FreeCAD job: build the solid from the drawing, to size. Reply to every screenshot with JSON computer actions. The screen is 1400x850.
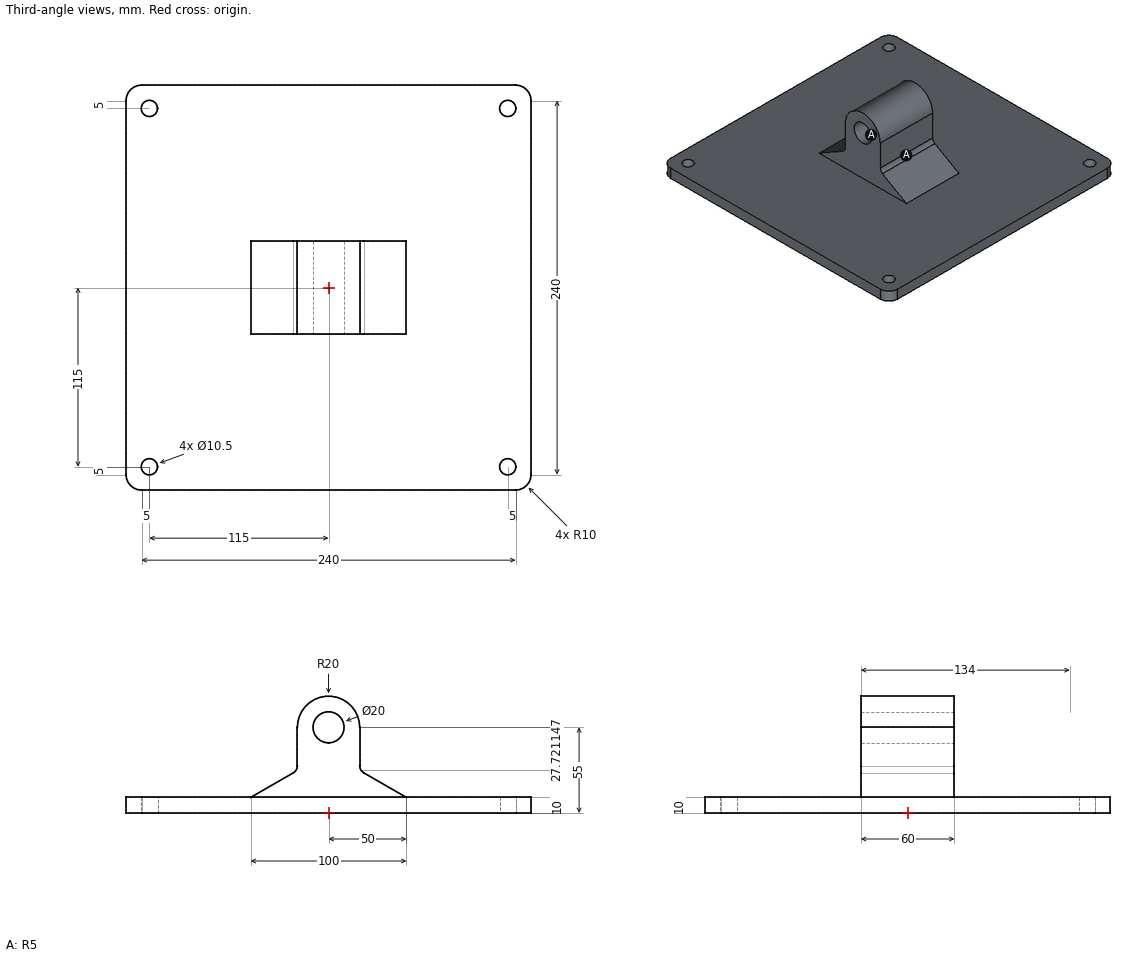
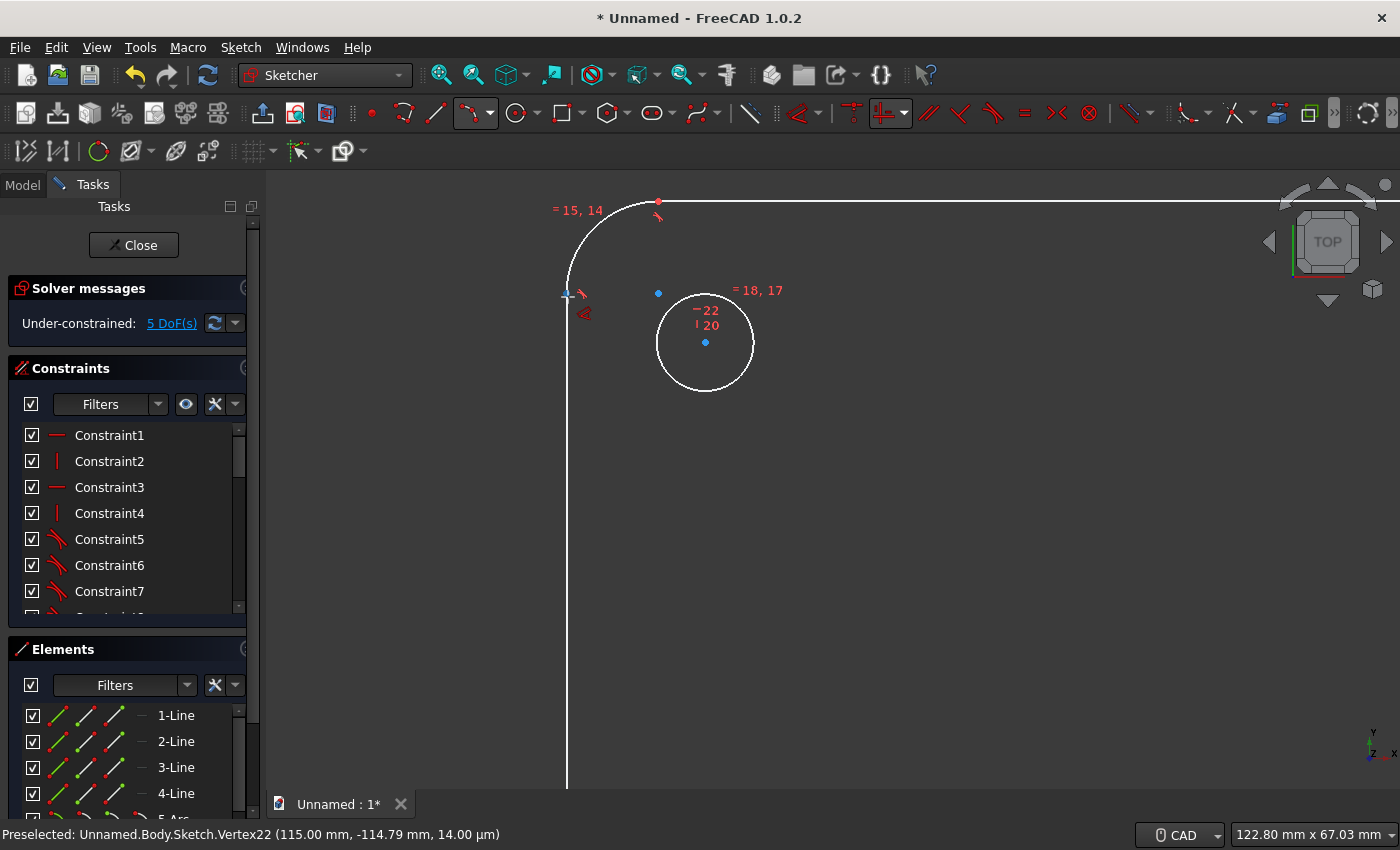
{"action": "left_click", "coordinate": [567, 294]}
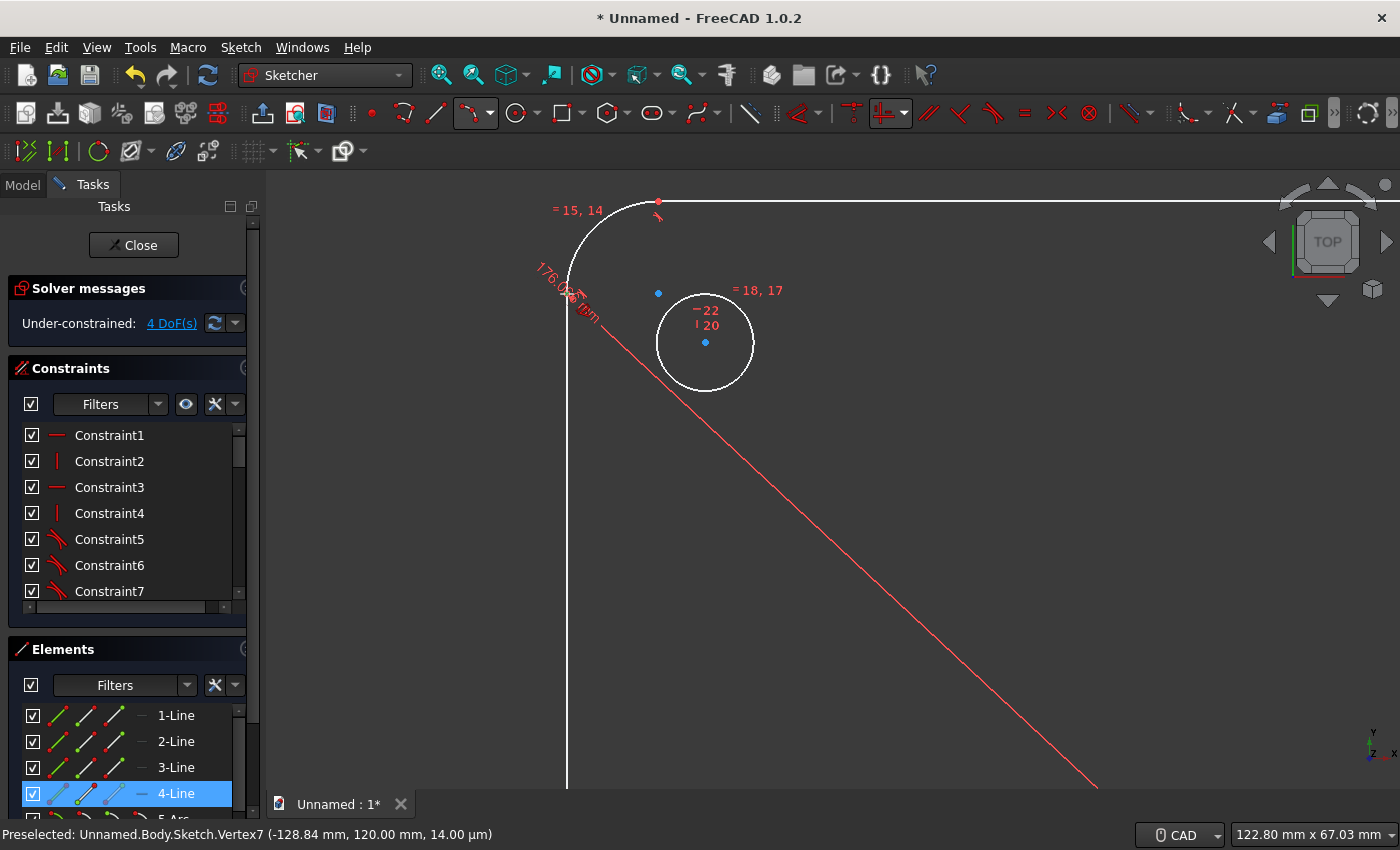
{"action": "left_click", "coordinate": [705, 343]}
{"action": "left_click", "coordinate": [533, 318]}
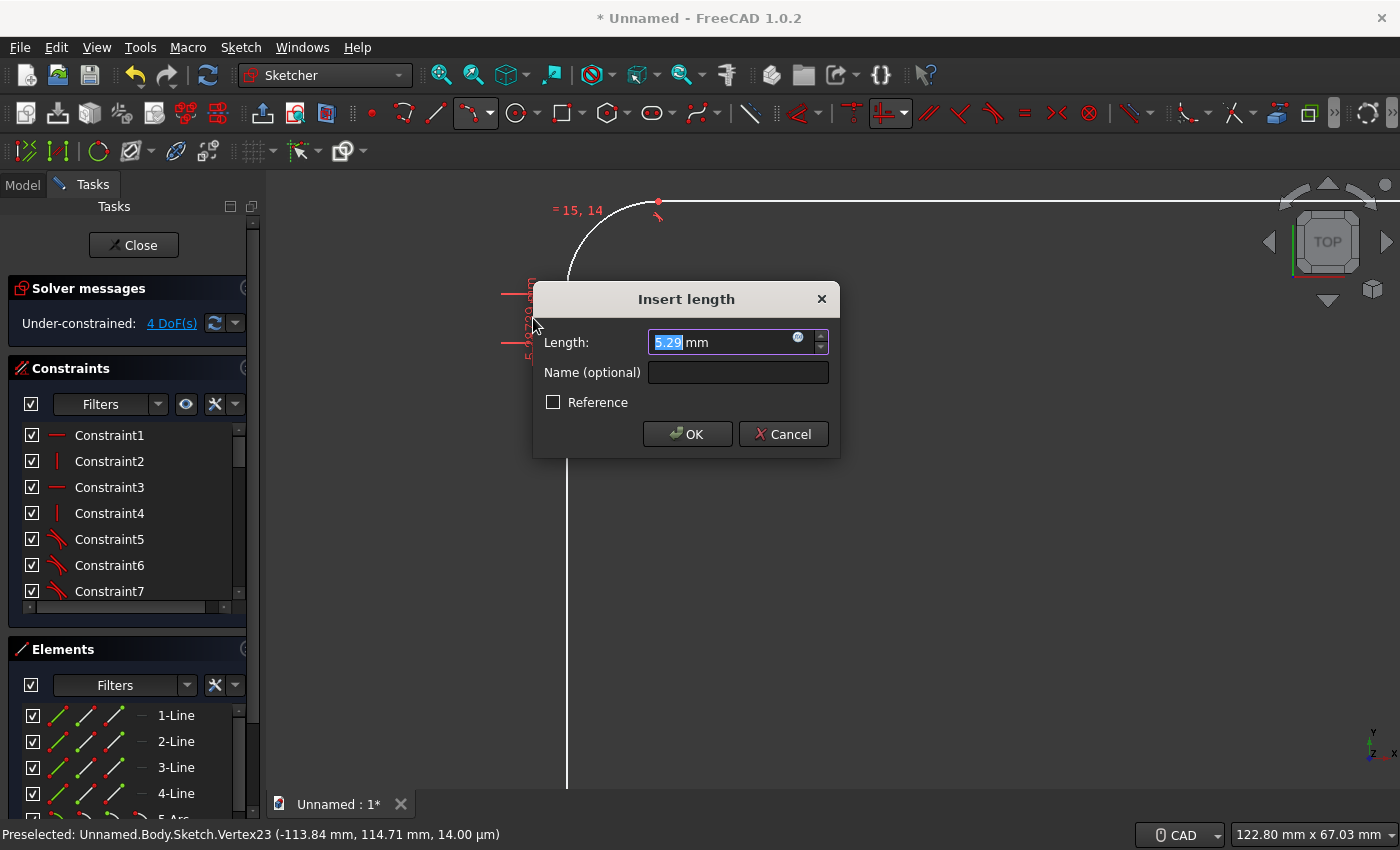
{"action": "type", "text": "5"}
{"action": "key", "text": "Return"}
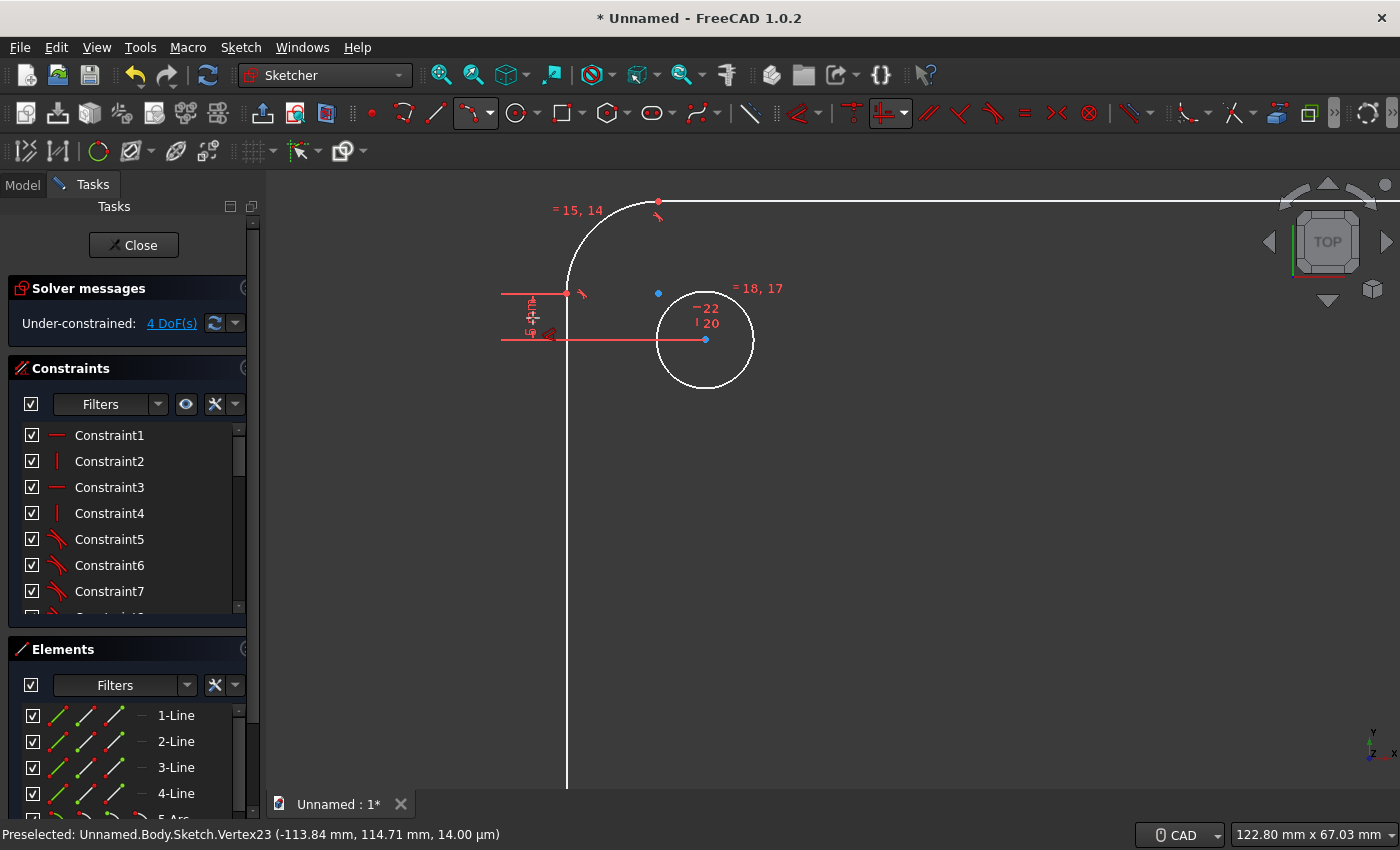
{"action": "scroll", "coordinate": [568, 297], "scroll_direction": "down", "scroll_amount": 9}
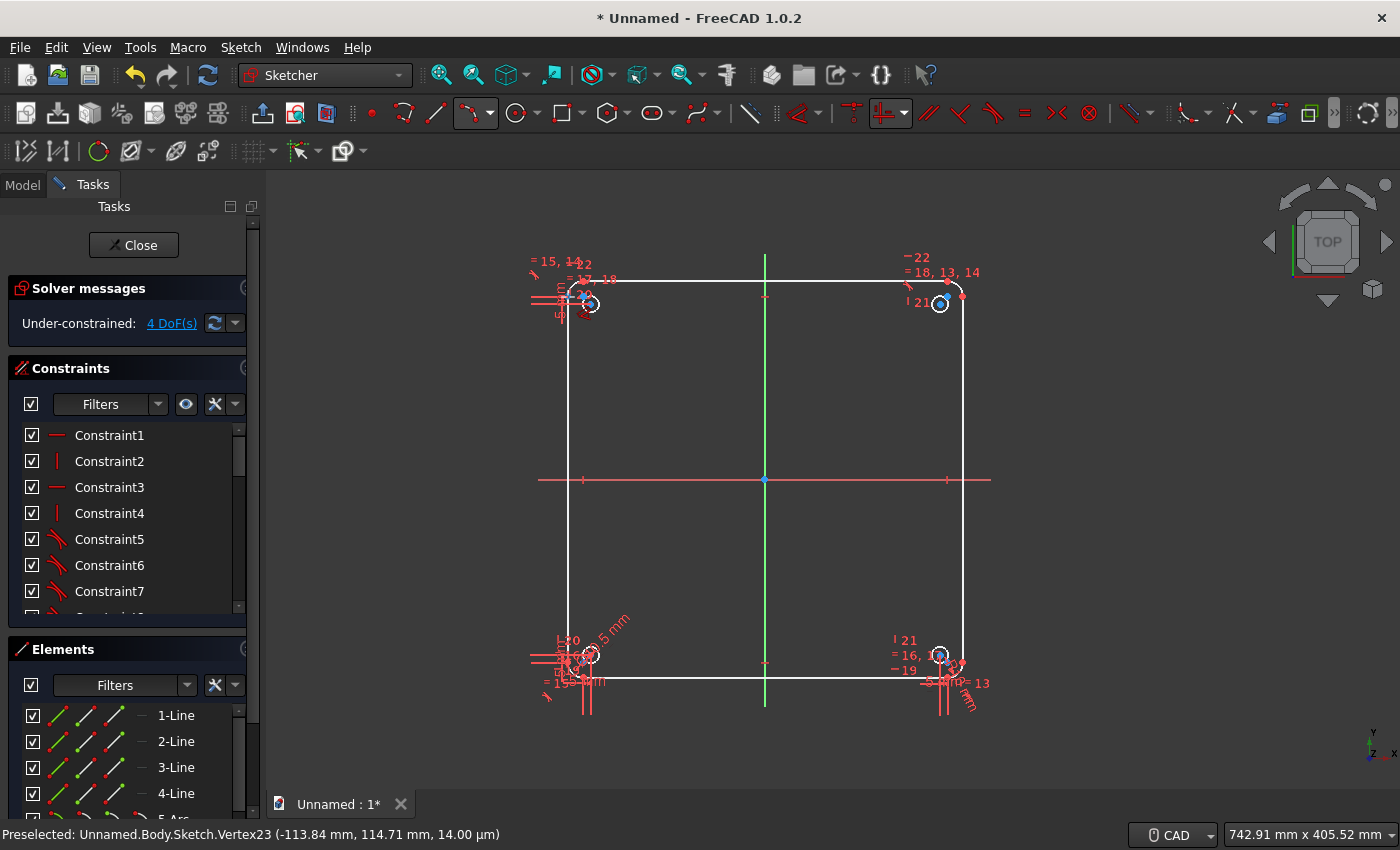
{"action": "left_click", "coordinate": [693, 678]}
{"action": "left_click", "coordinate": [682, 712]}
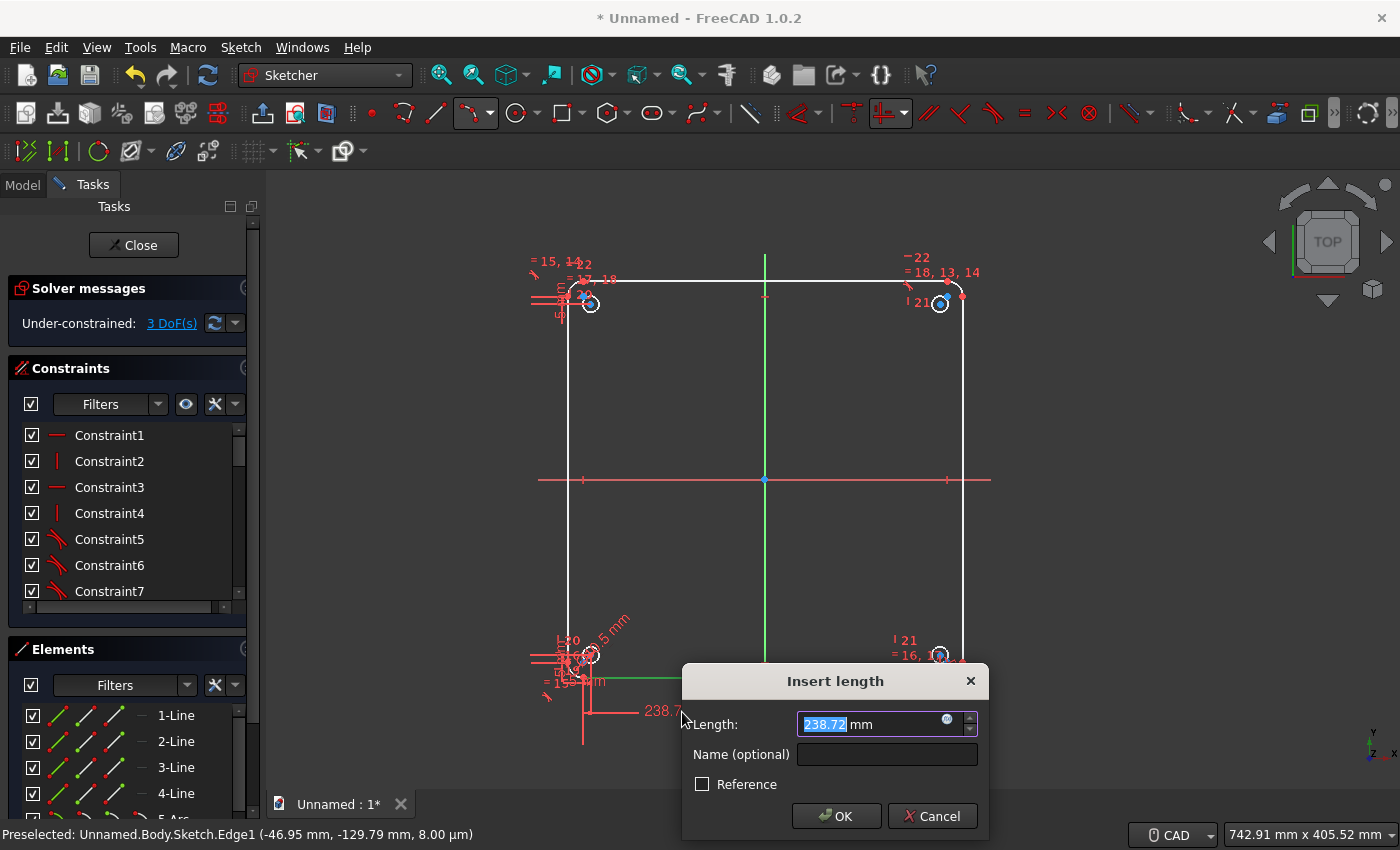
{"action": "type", "text": "240"}
{"action": "key", "text": "Return"}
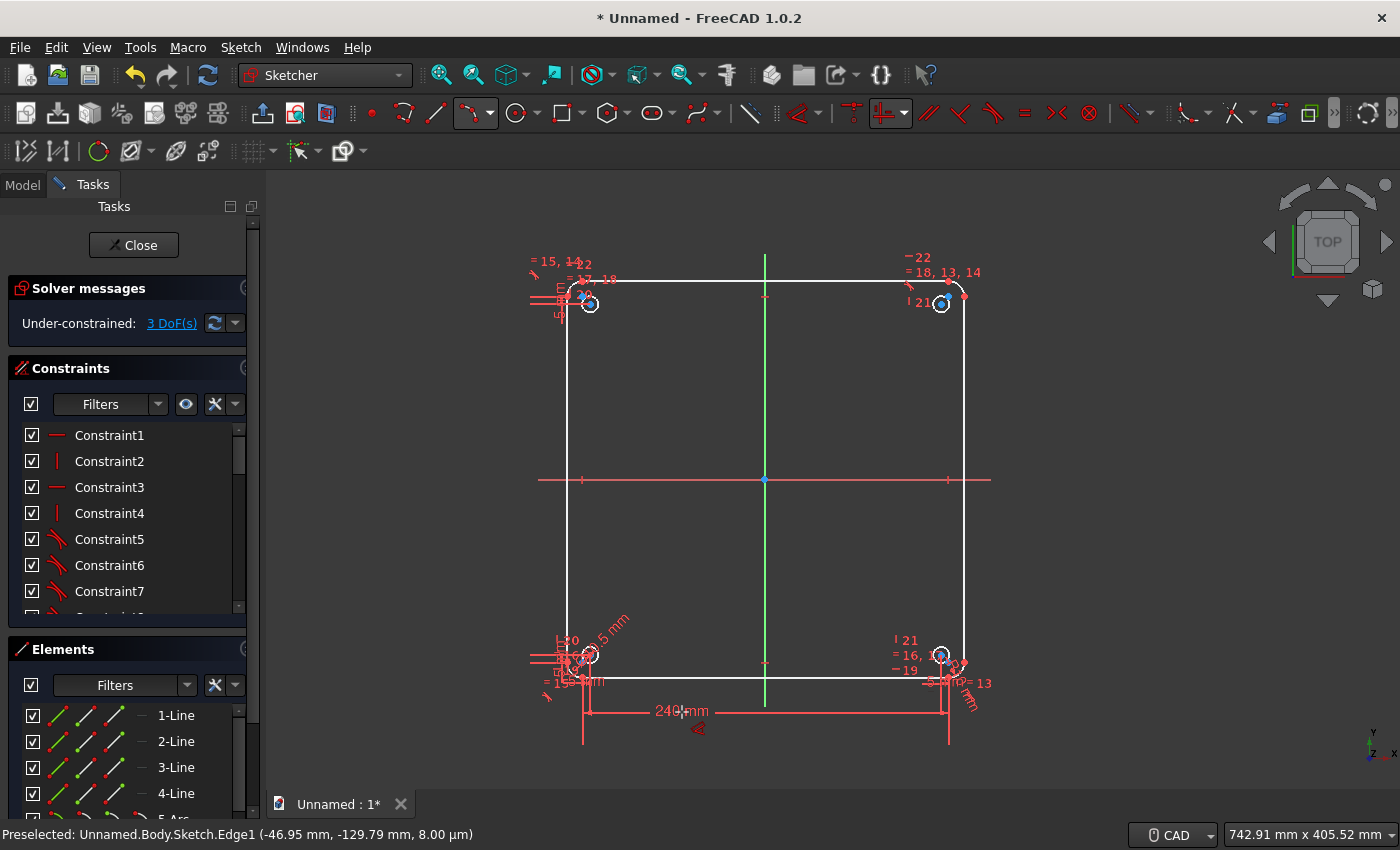
{"action": "left_click", "coordinate": [964, 553]}
{"action": "left_click", "coordinate": [998, 395]}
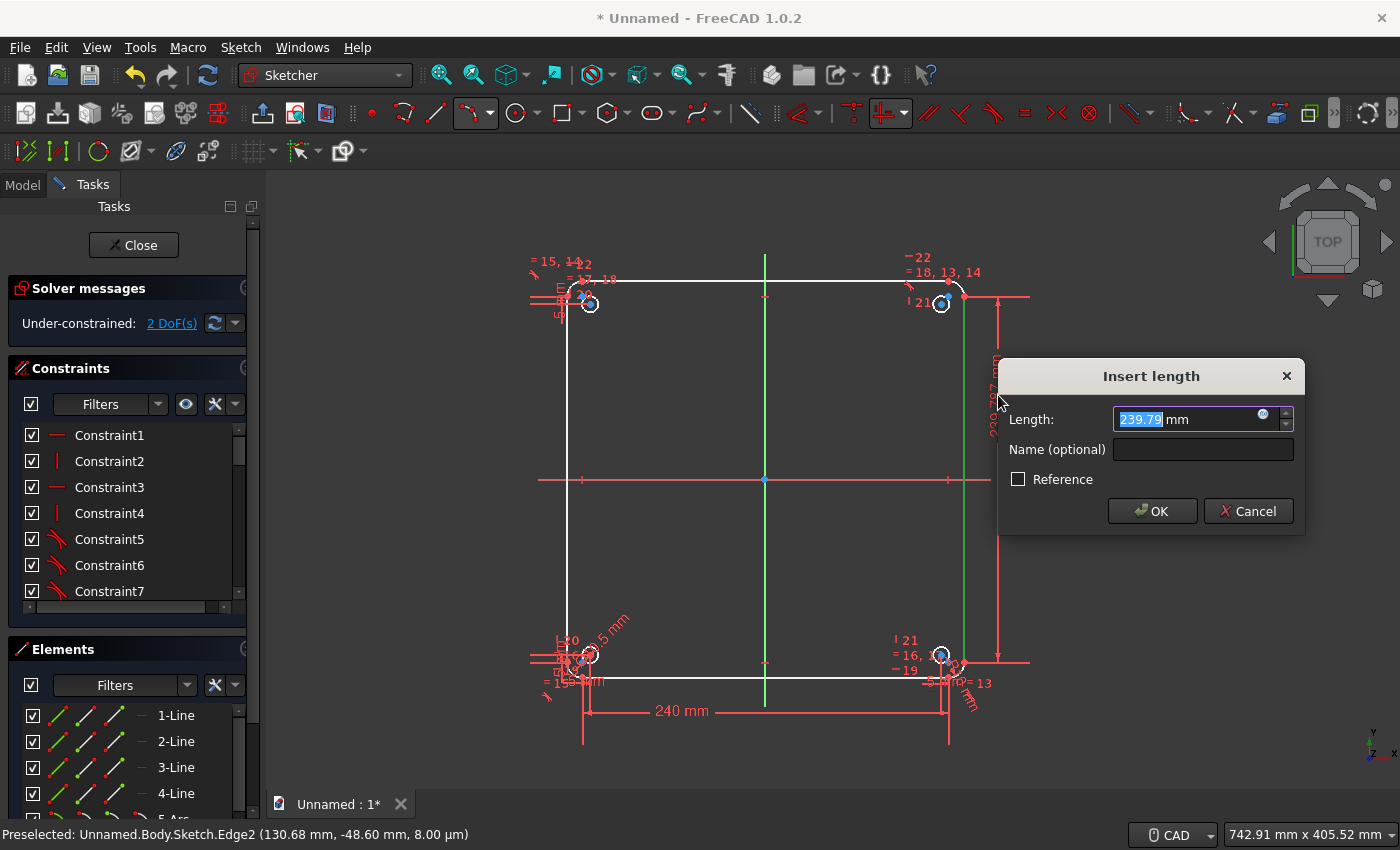
{"action": "type", "text": "240"}
{"action": "key", "text": "Return"}